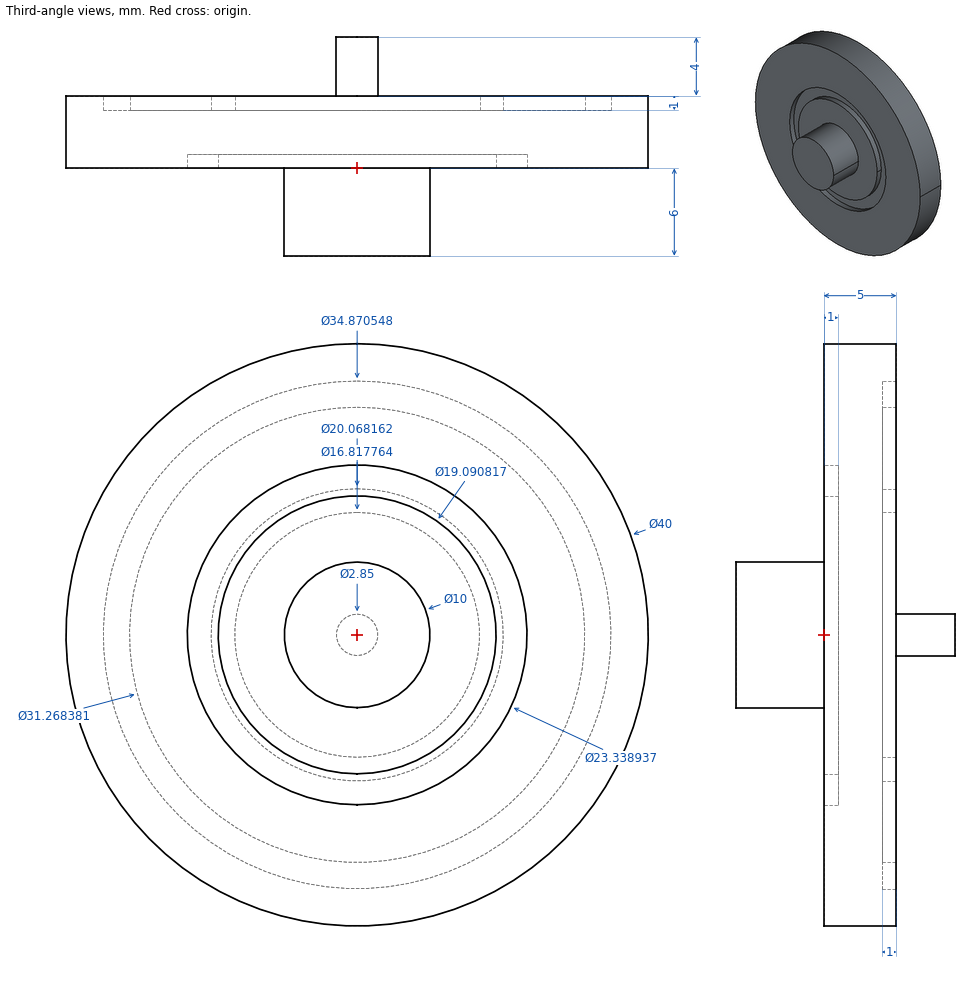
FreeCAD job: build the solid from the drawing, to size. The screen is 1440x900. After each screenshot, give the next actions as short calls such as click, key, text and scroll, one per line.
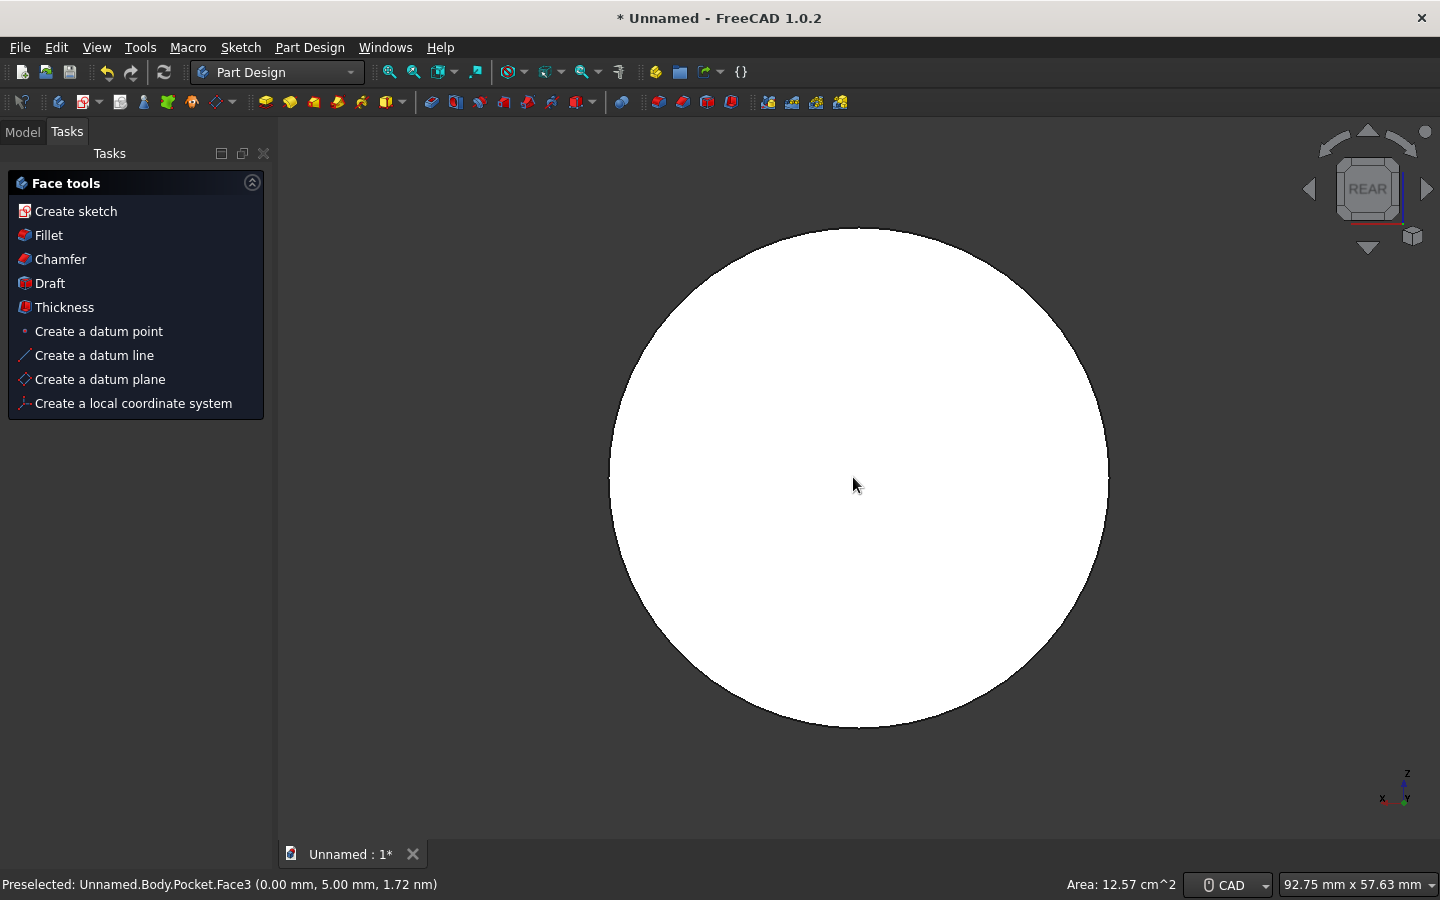
click(84, 102)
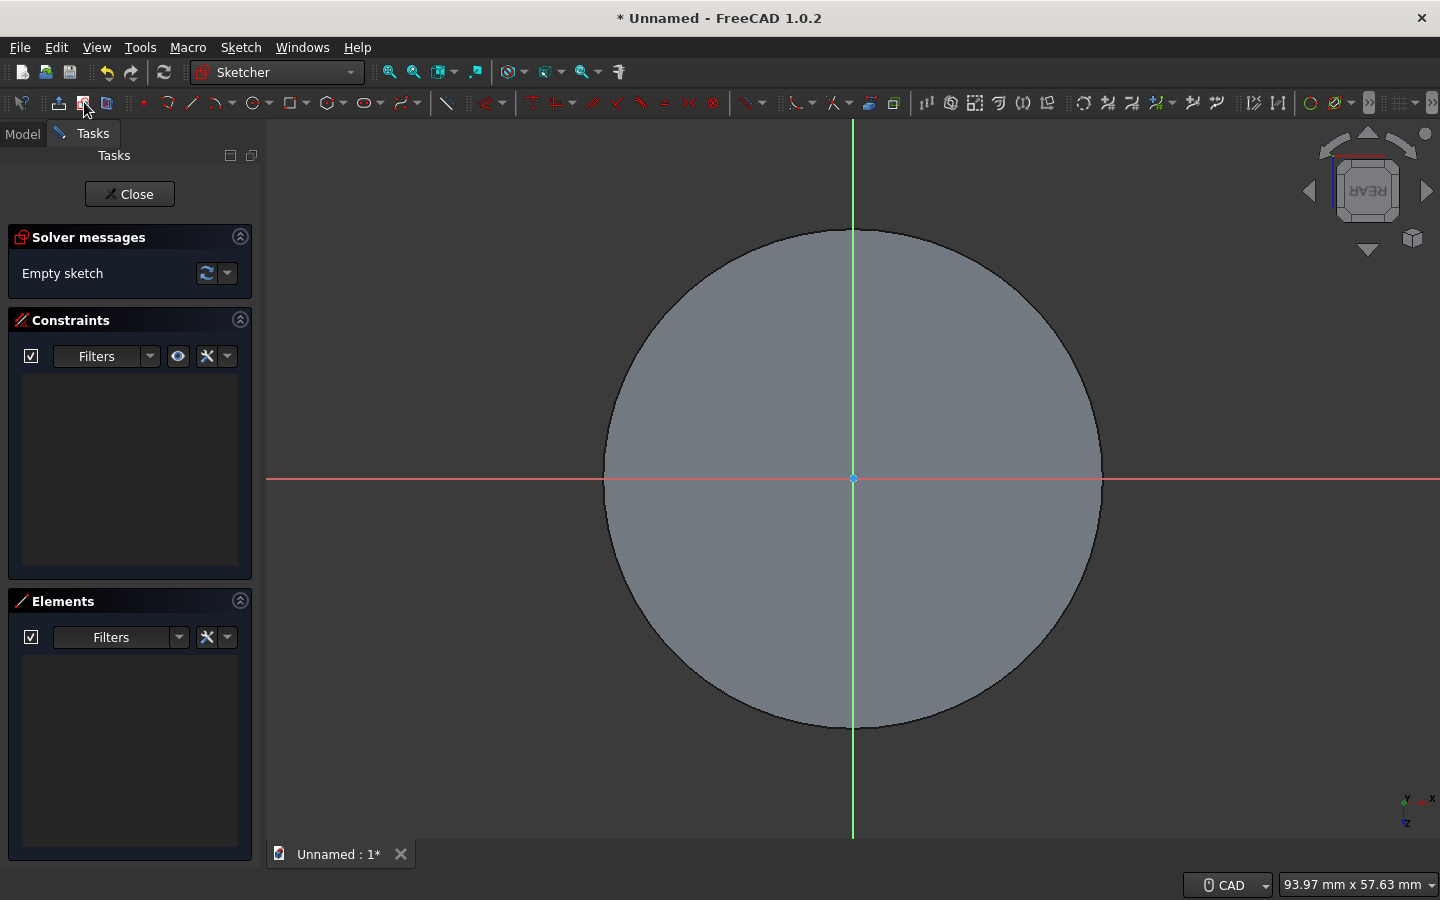
scroll(858, 479, up, 13)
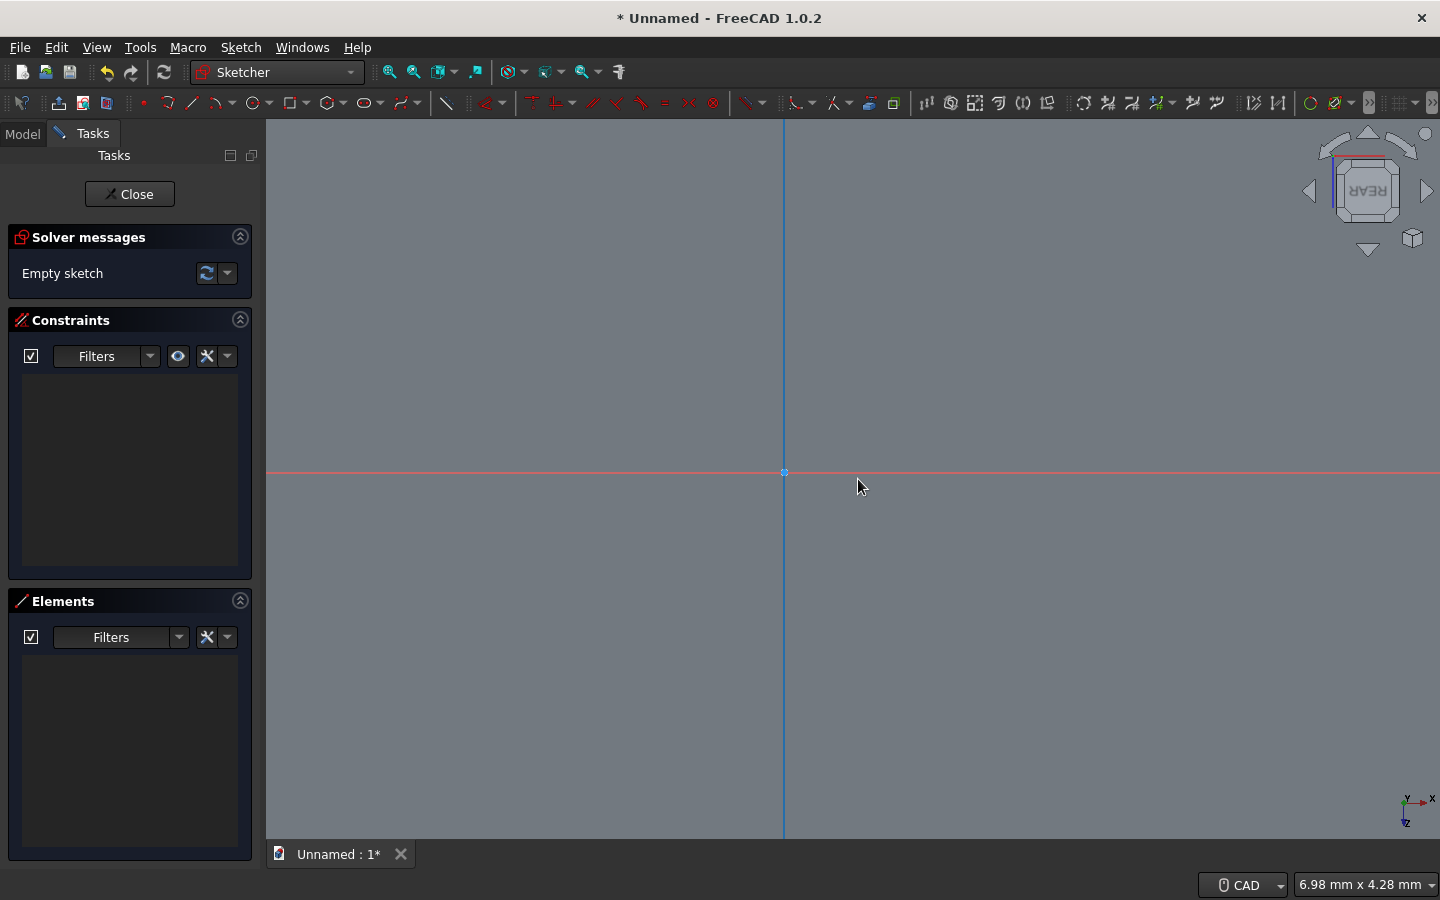
key(g)
key(c)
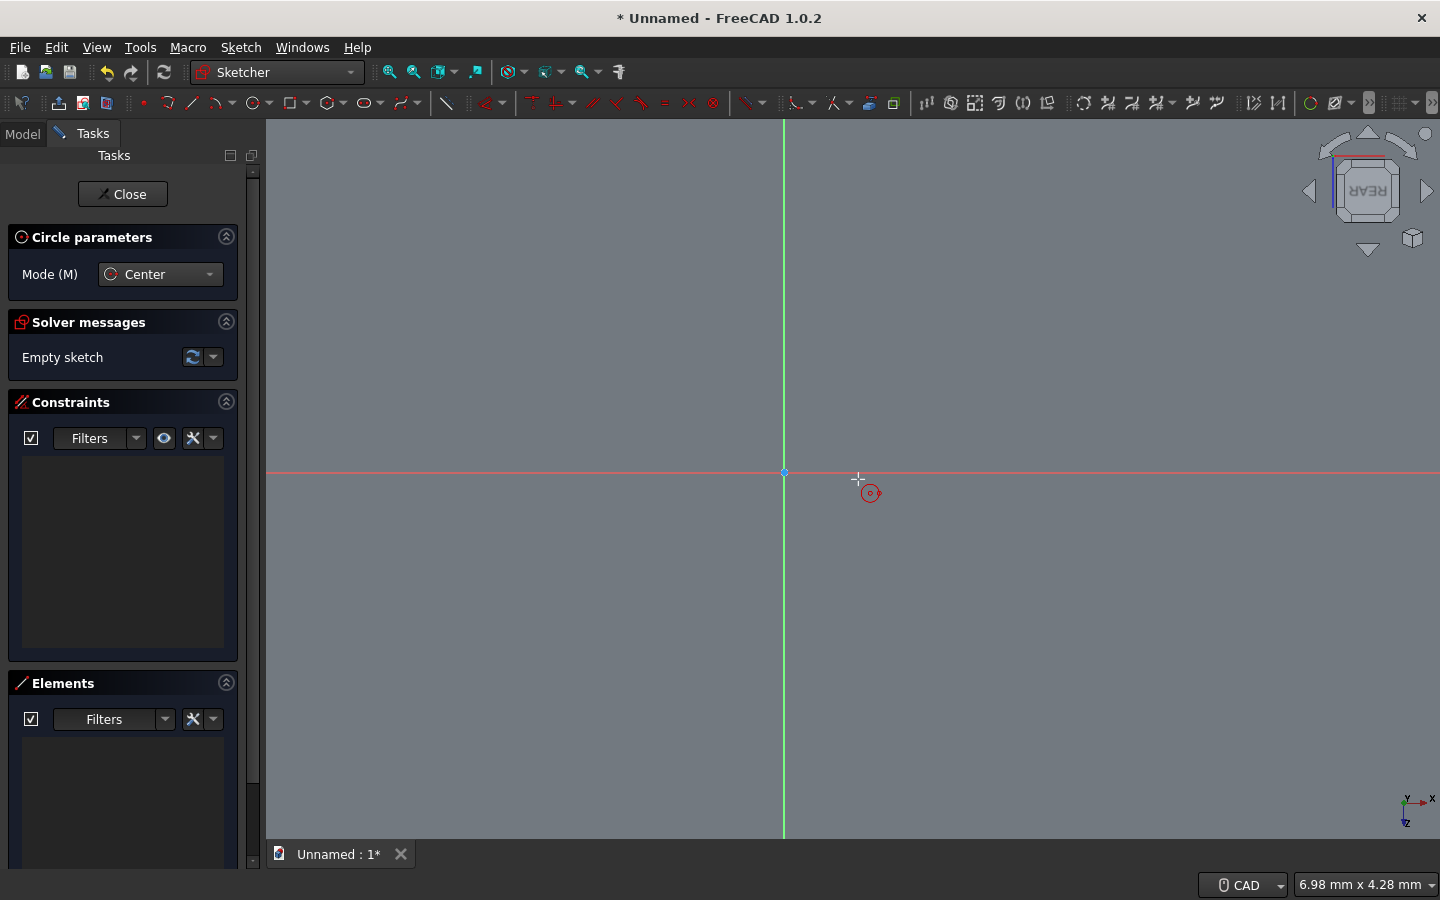
click(784, 473)
click(954, 303)
key(Escape)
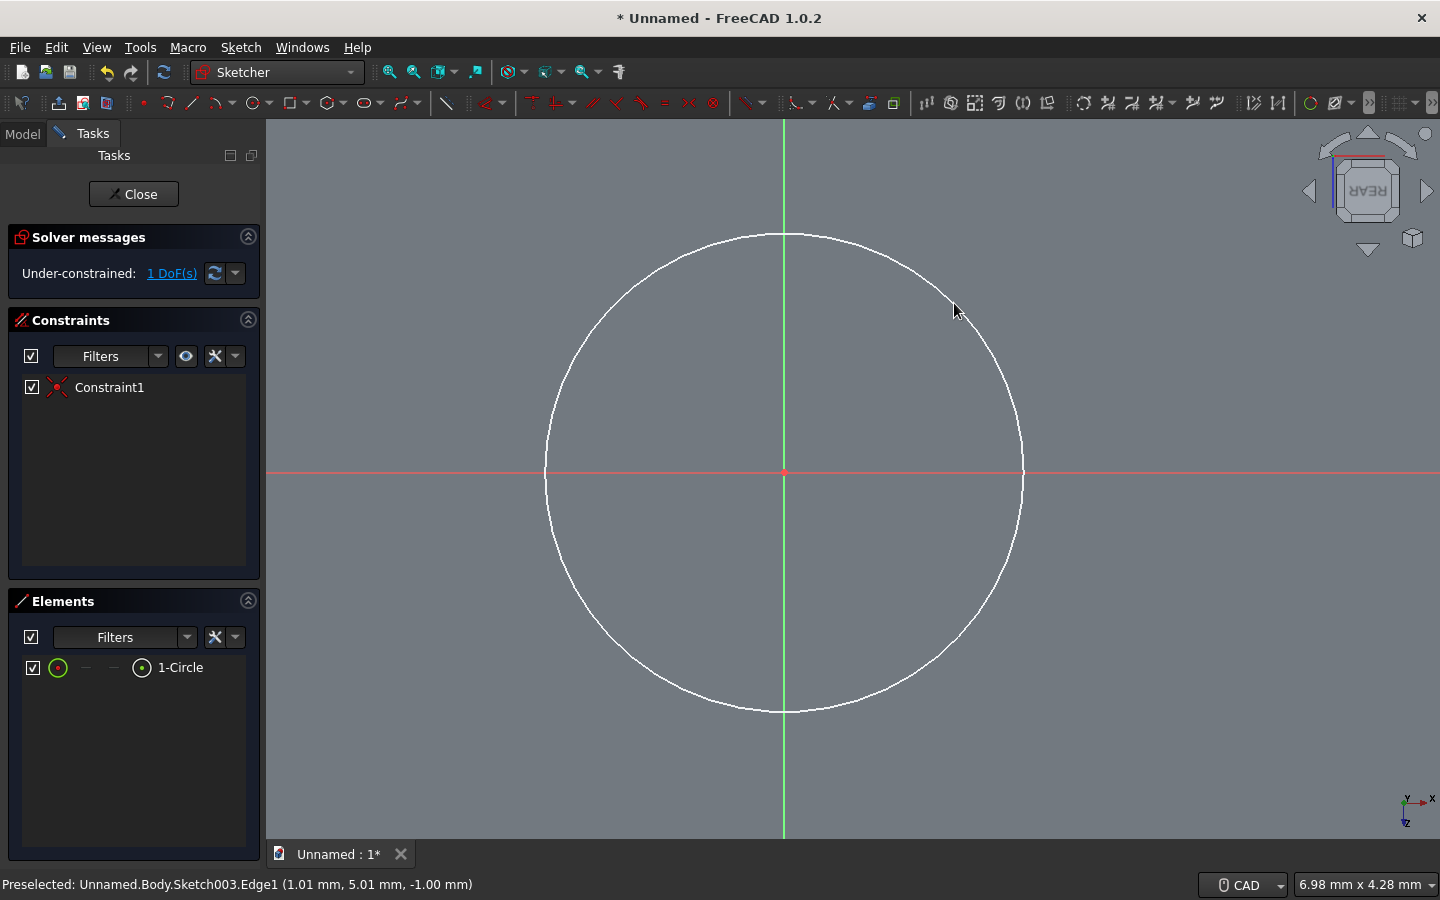
click(486, 104)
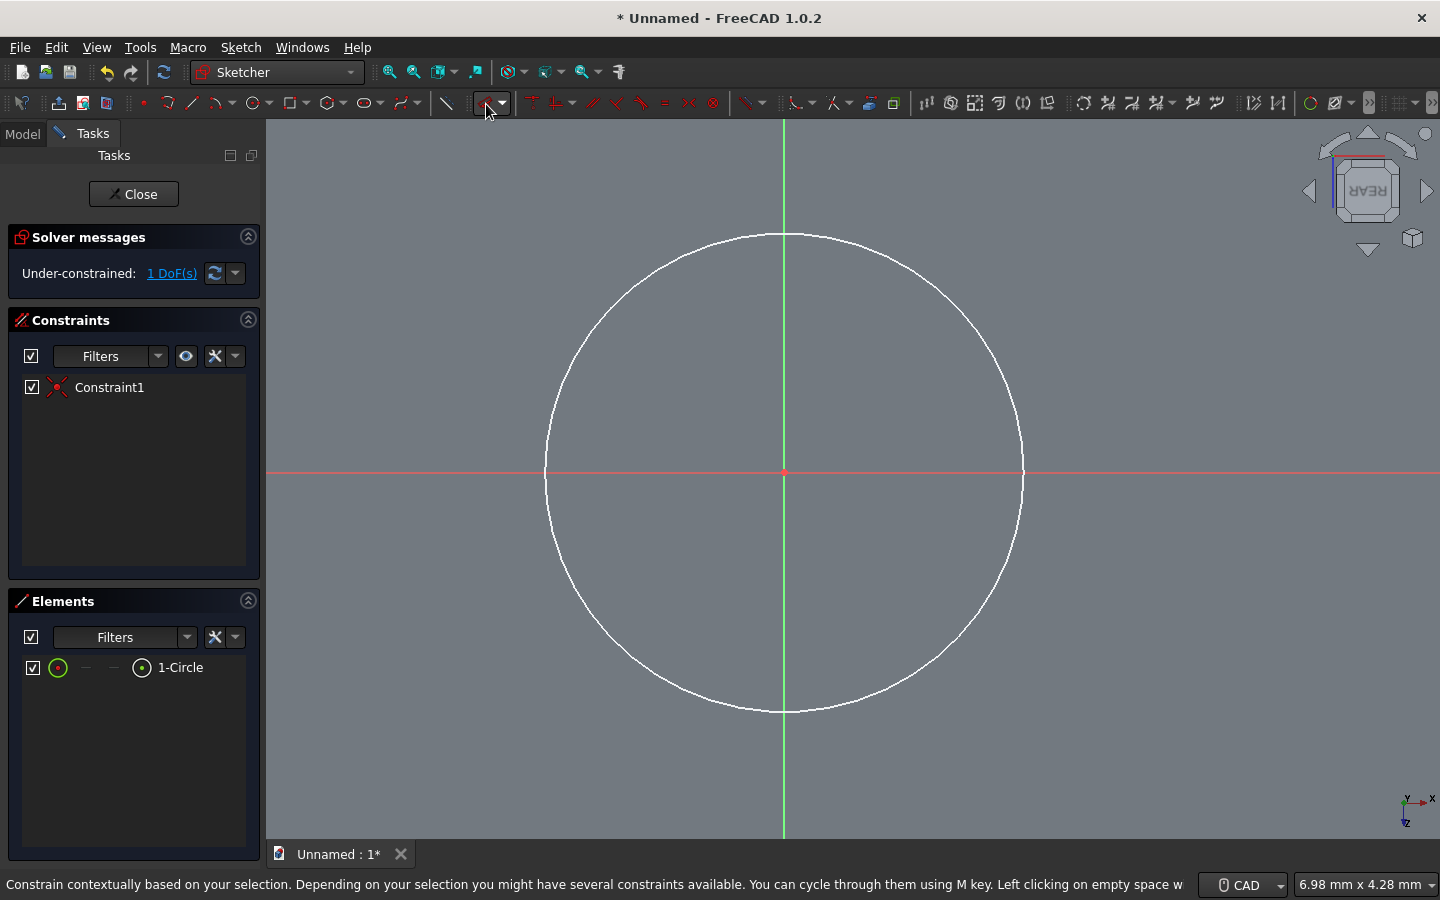
click(953, 303)
click(976, 280)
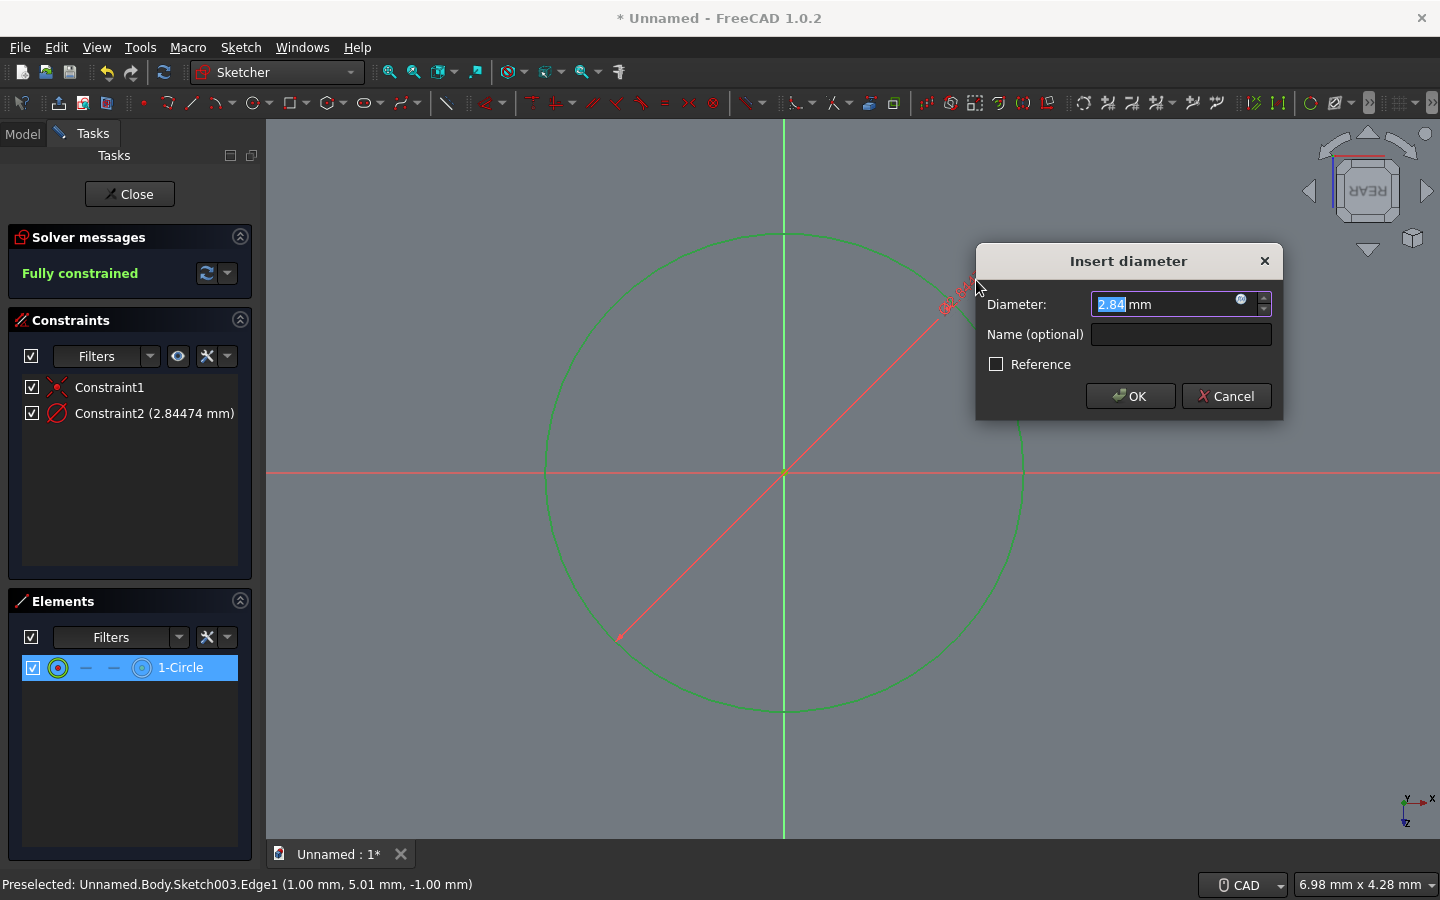
text(2.85)
key(Return)
key(Escape)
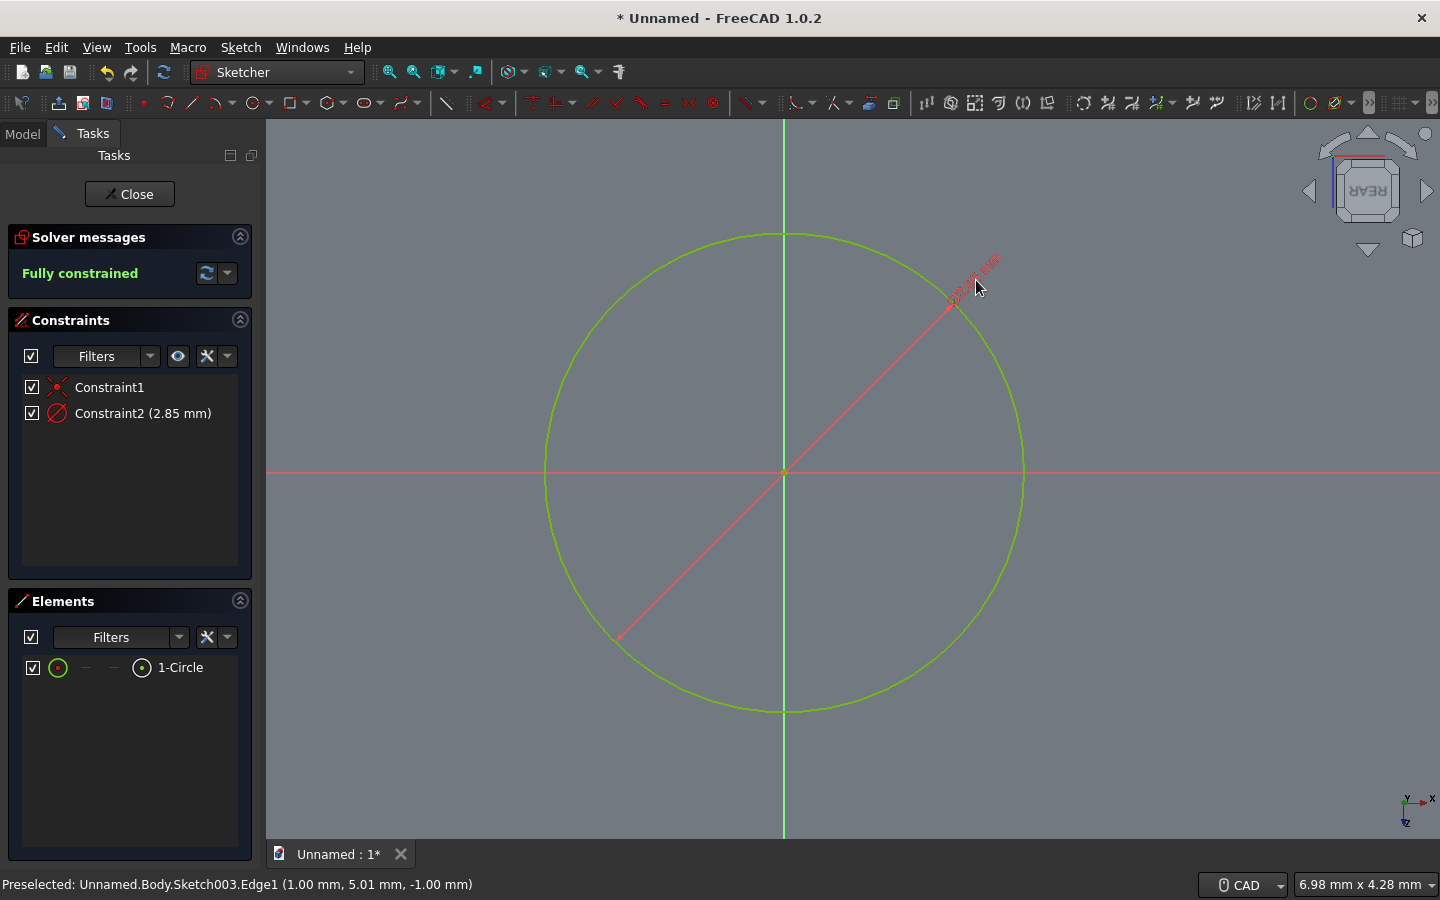
click(130, 194)